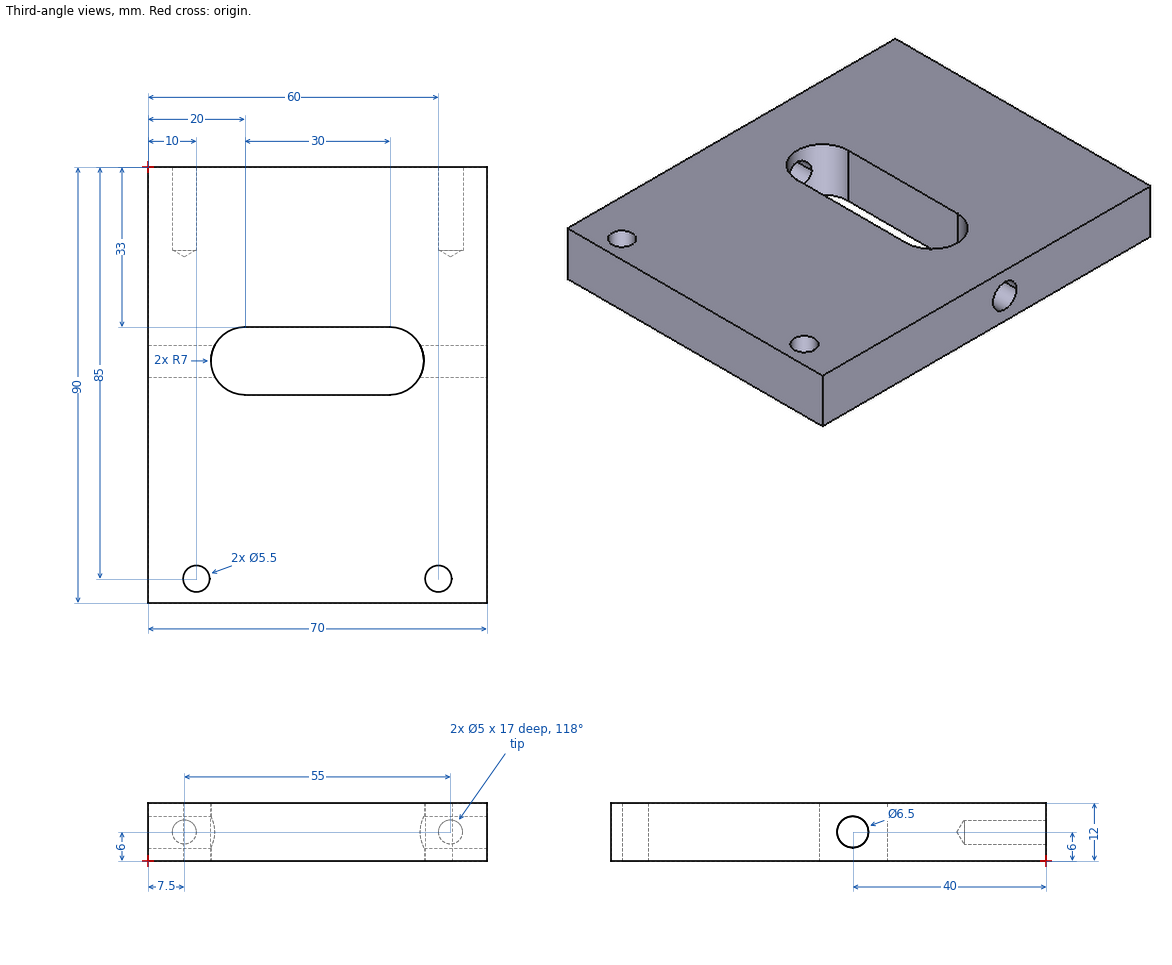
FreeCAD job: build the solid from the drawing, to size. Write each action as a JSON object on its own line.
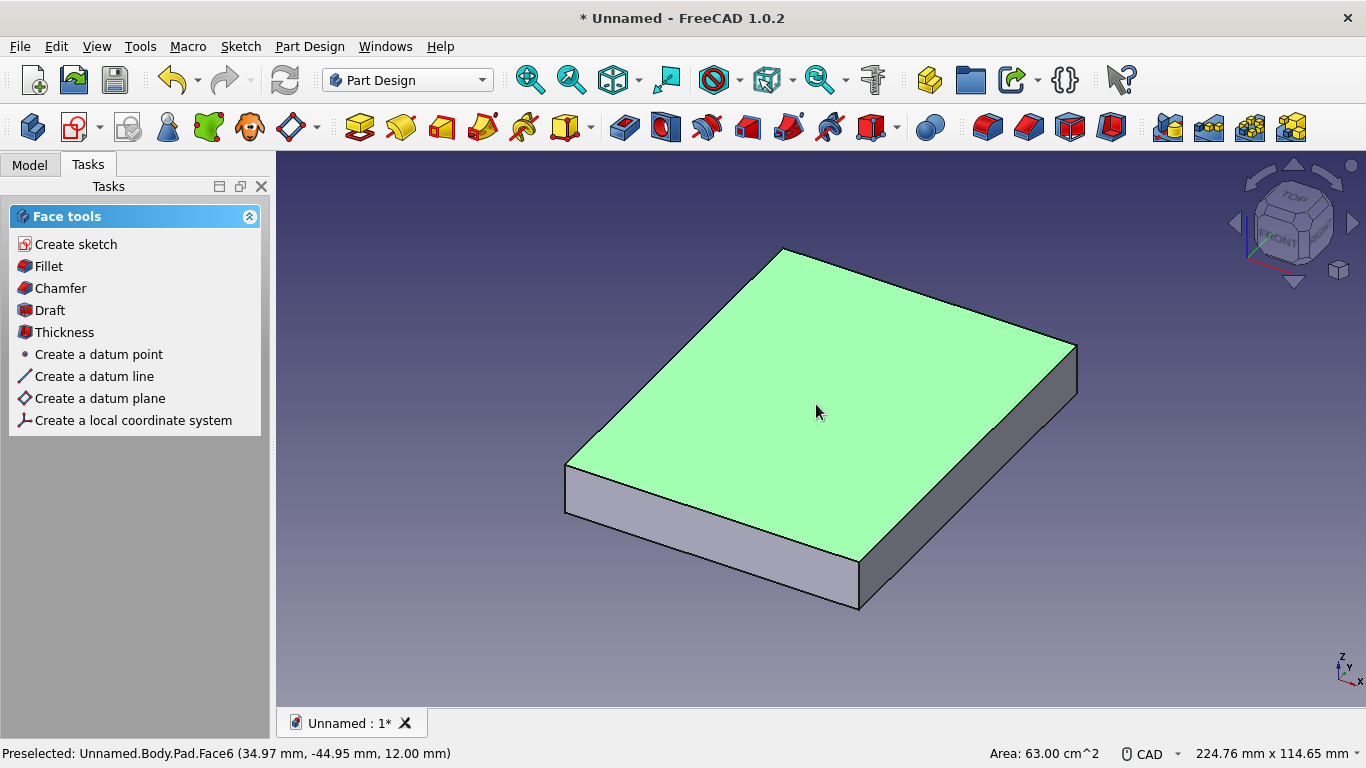
{"action": "left_click", "coordinate": [74, 128]}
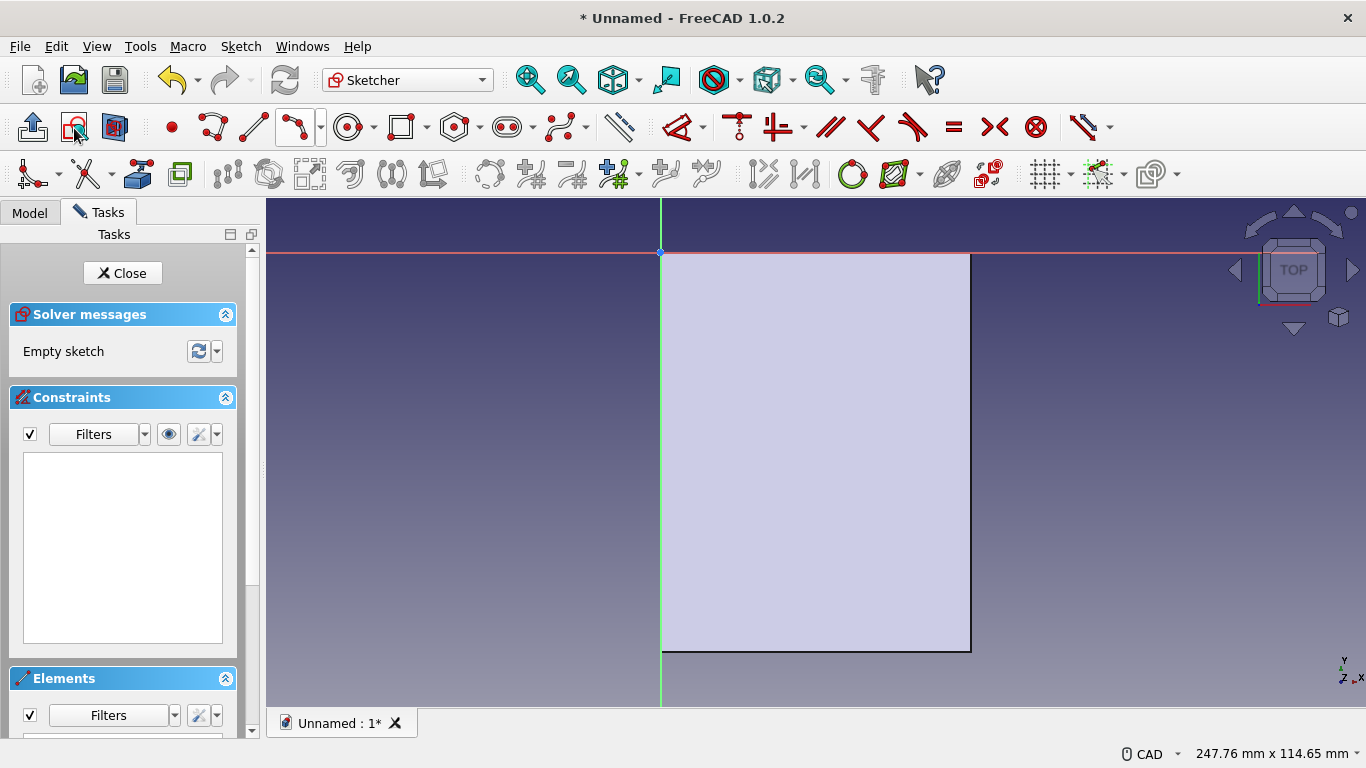
{"action": "scroll", "coordinate": [868, 226], "scroll_direction": "up", "scroll_amount": 2}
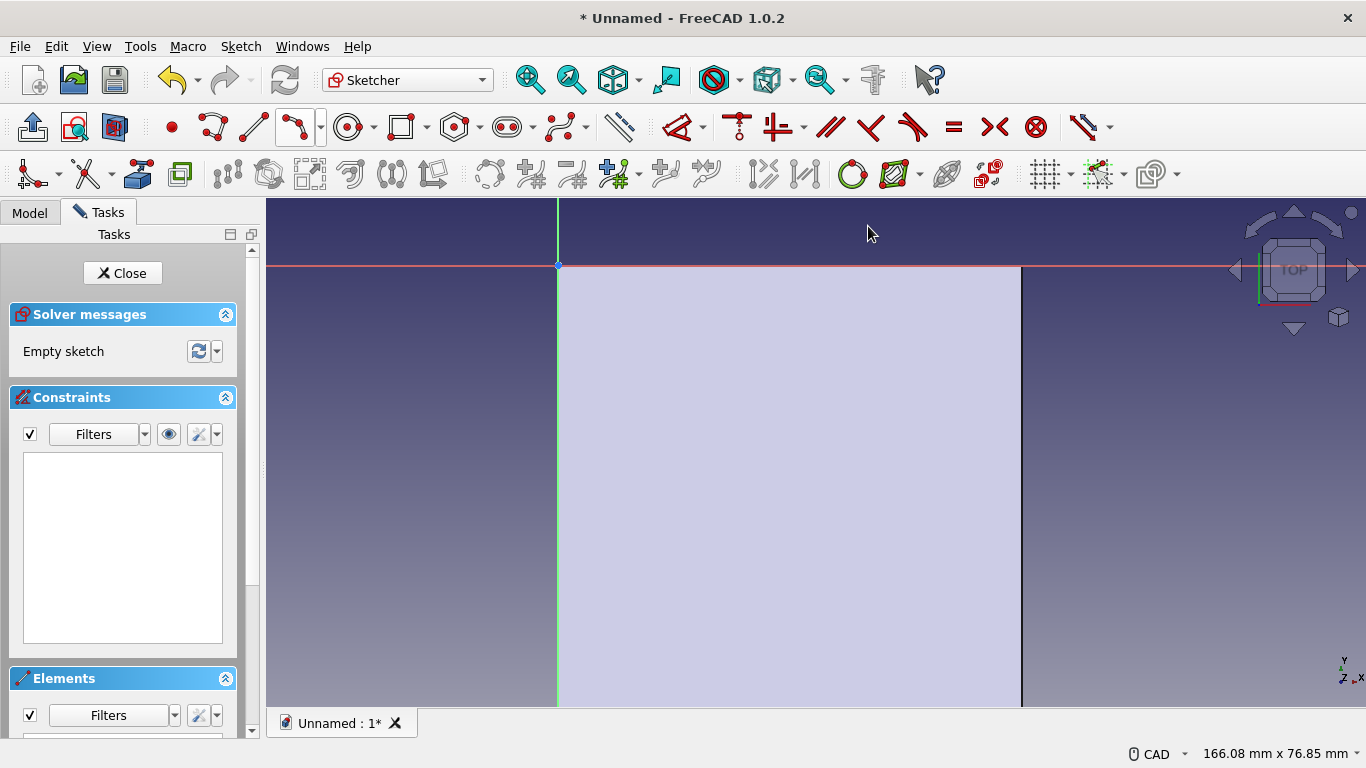
{"action": "left_click", "coordinate": [506, 128]}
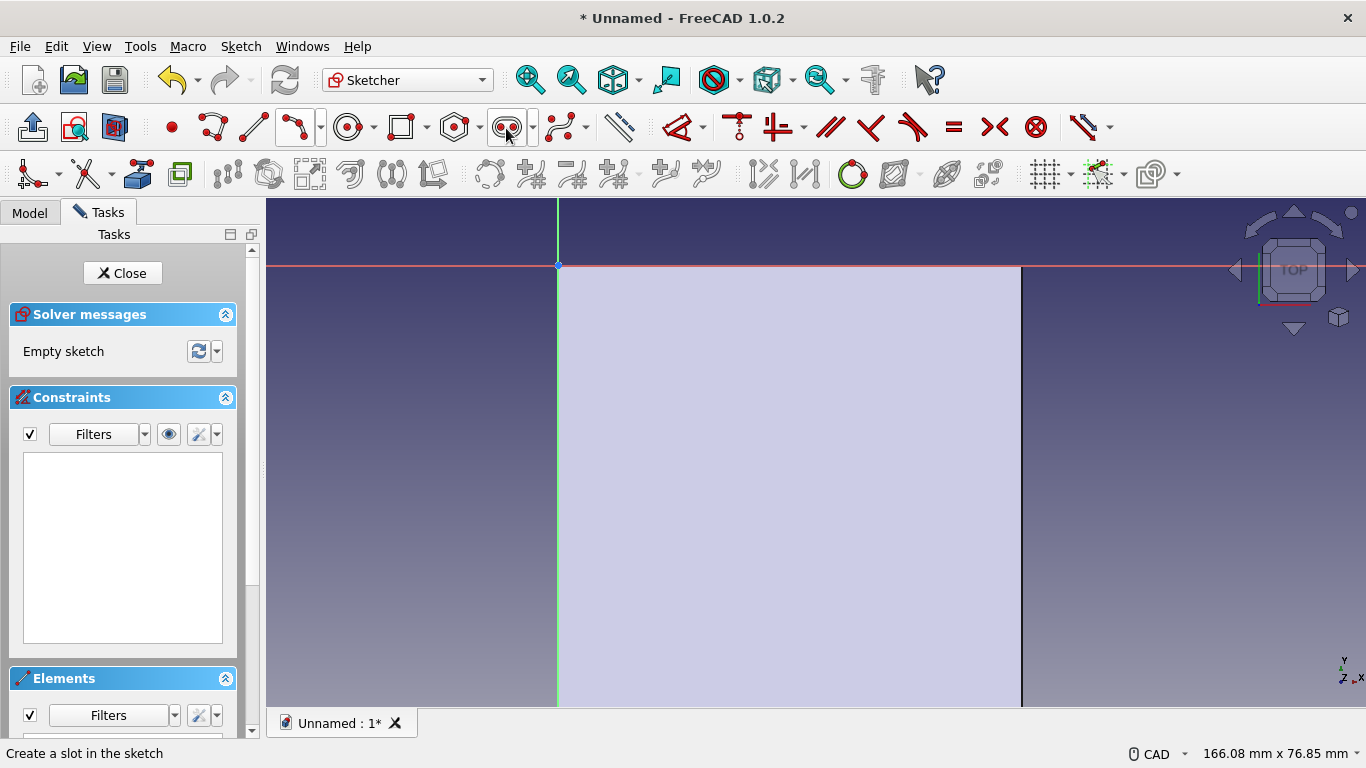
{"action": "left_click", "coordinate": [691, 531]}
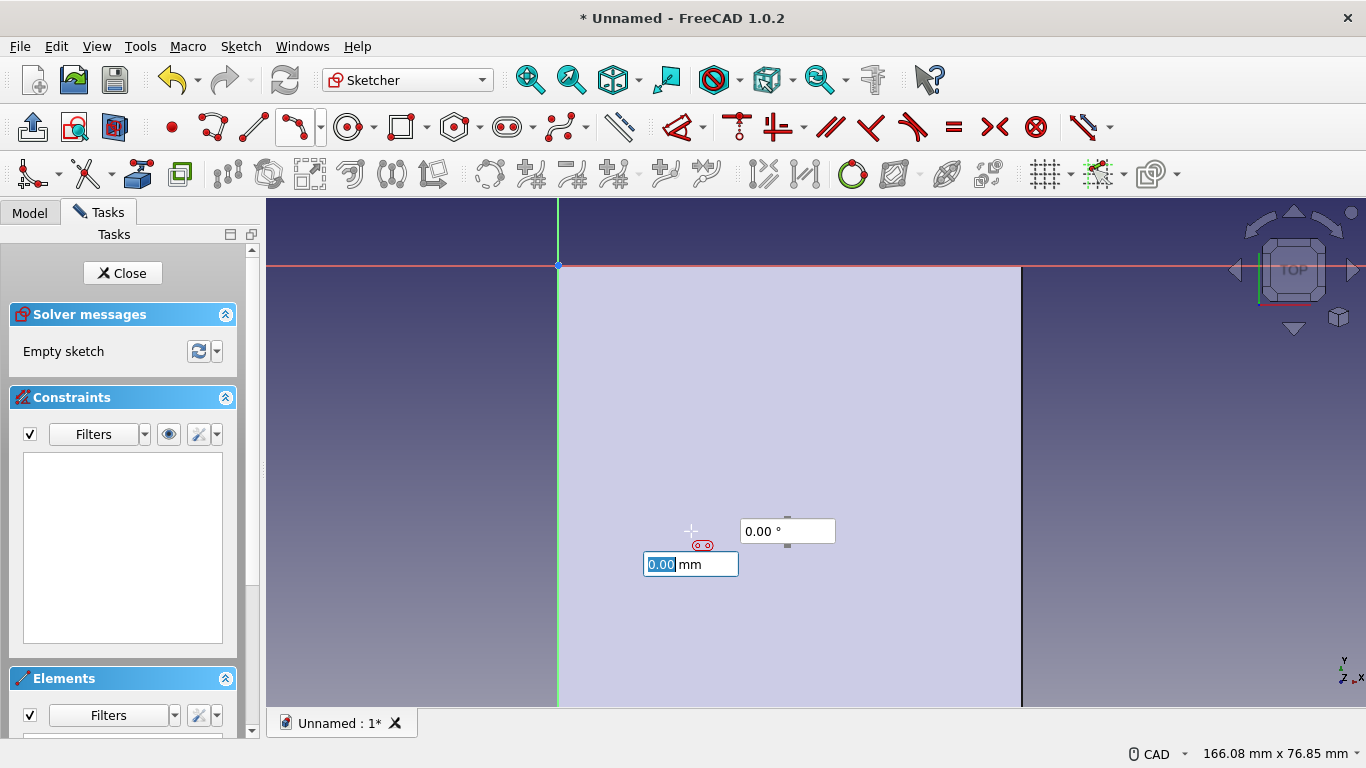
{"action": "left_click", "coordinate": [890, 531]}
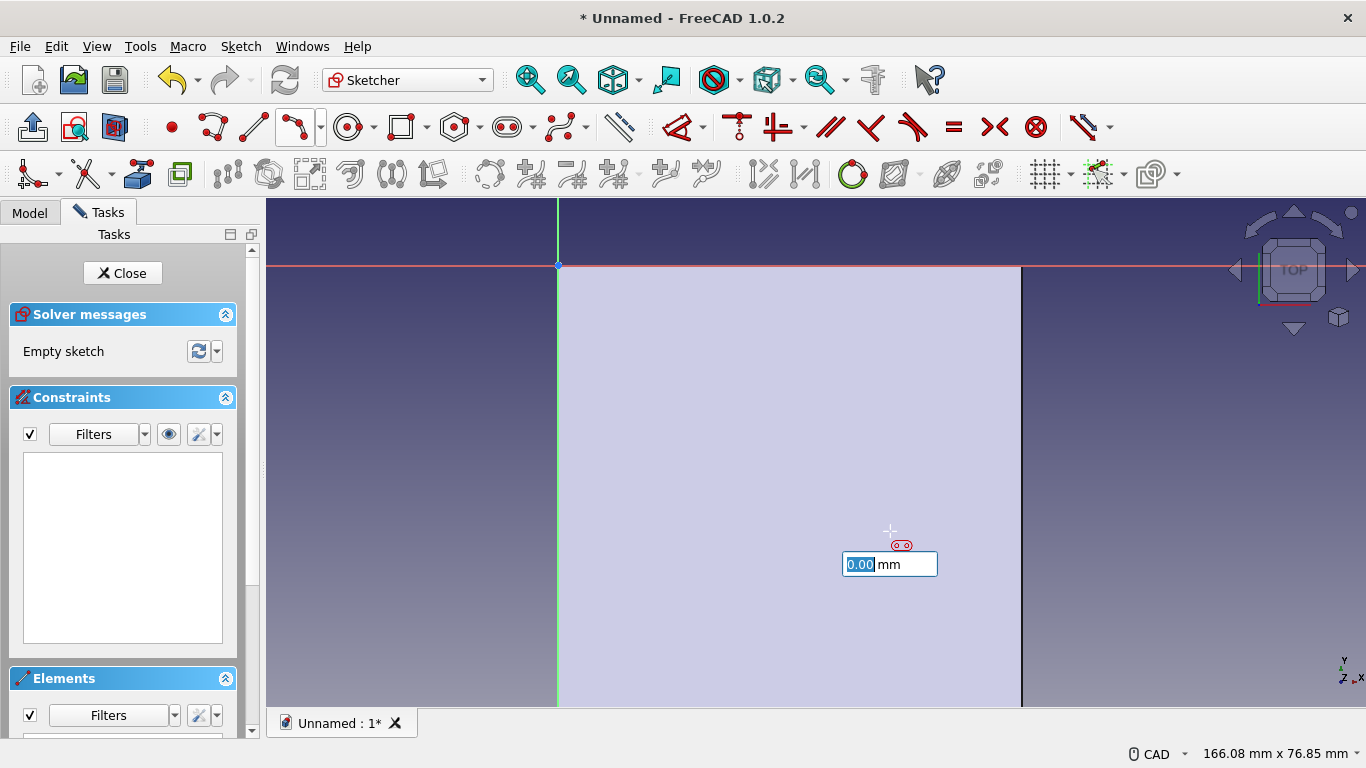
{"action": "left_click", "coordinate": [790, 484]}
{"action": "key", "text": "Escape"}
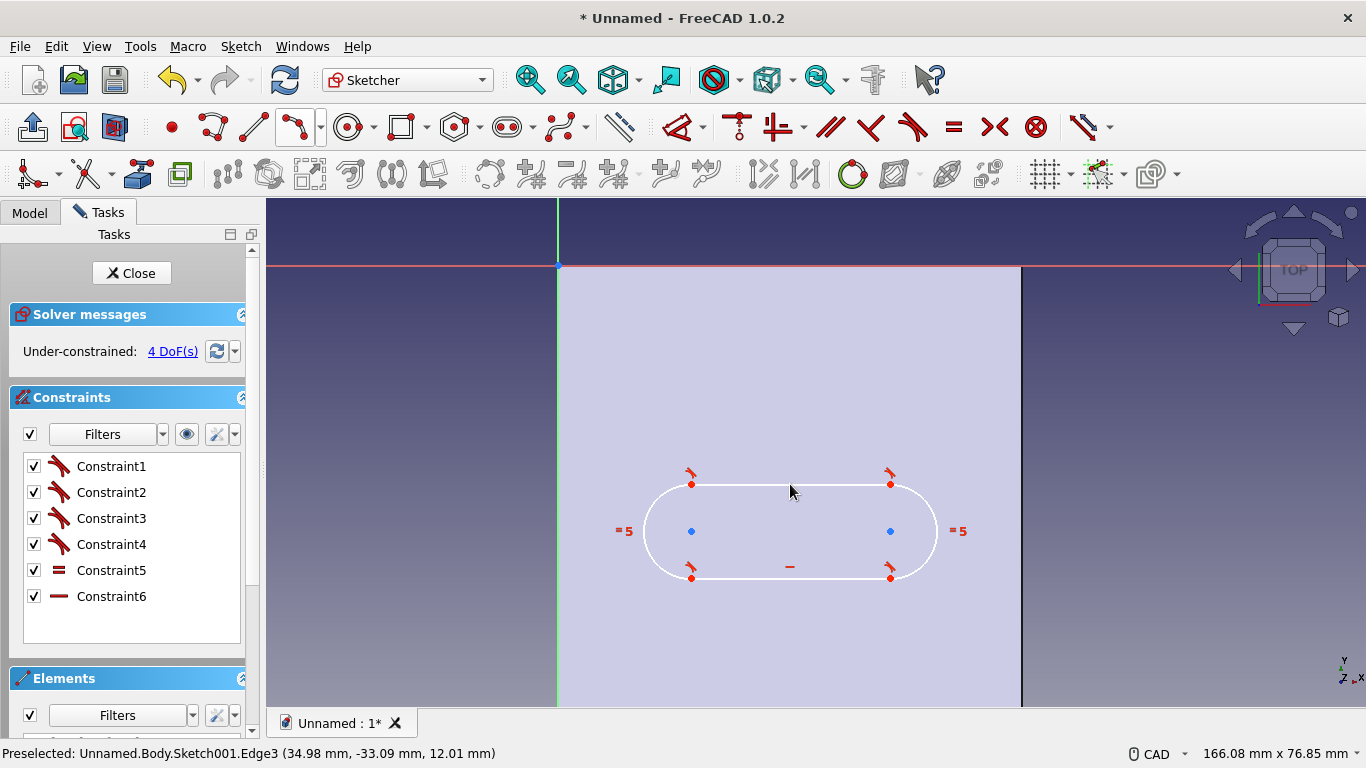
{"action": "left_click", "coordinate": [676, 128]}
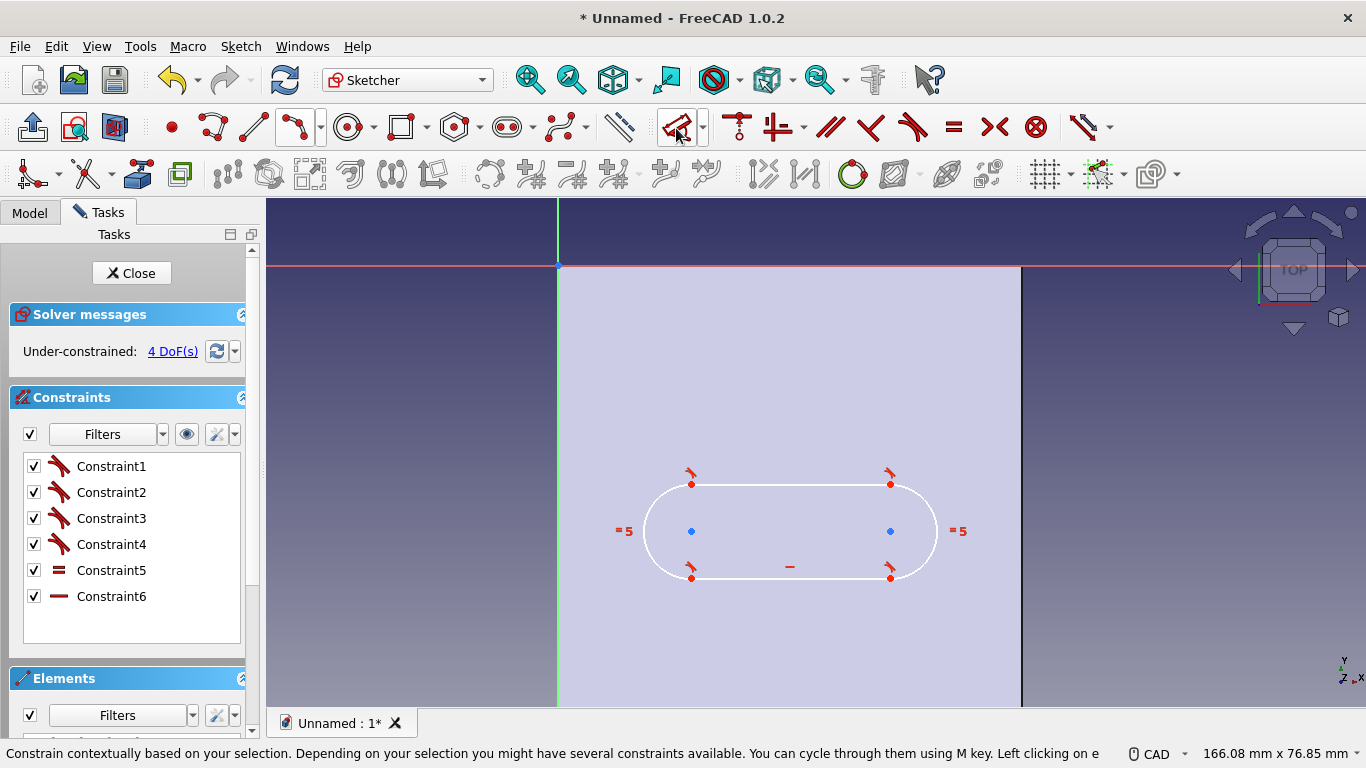
{"action": "left_click", "coordinate": [653, 504]}
{"action": "left_click", "coordinate": [627, 485]}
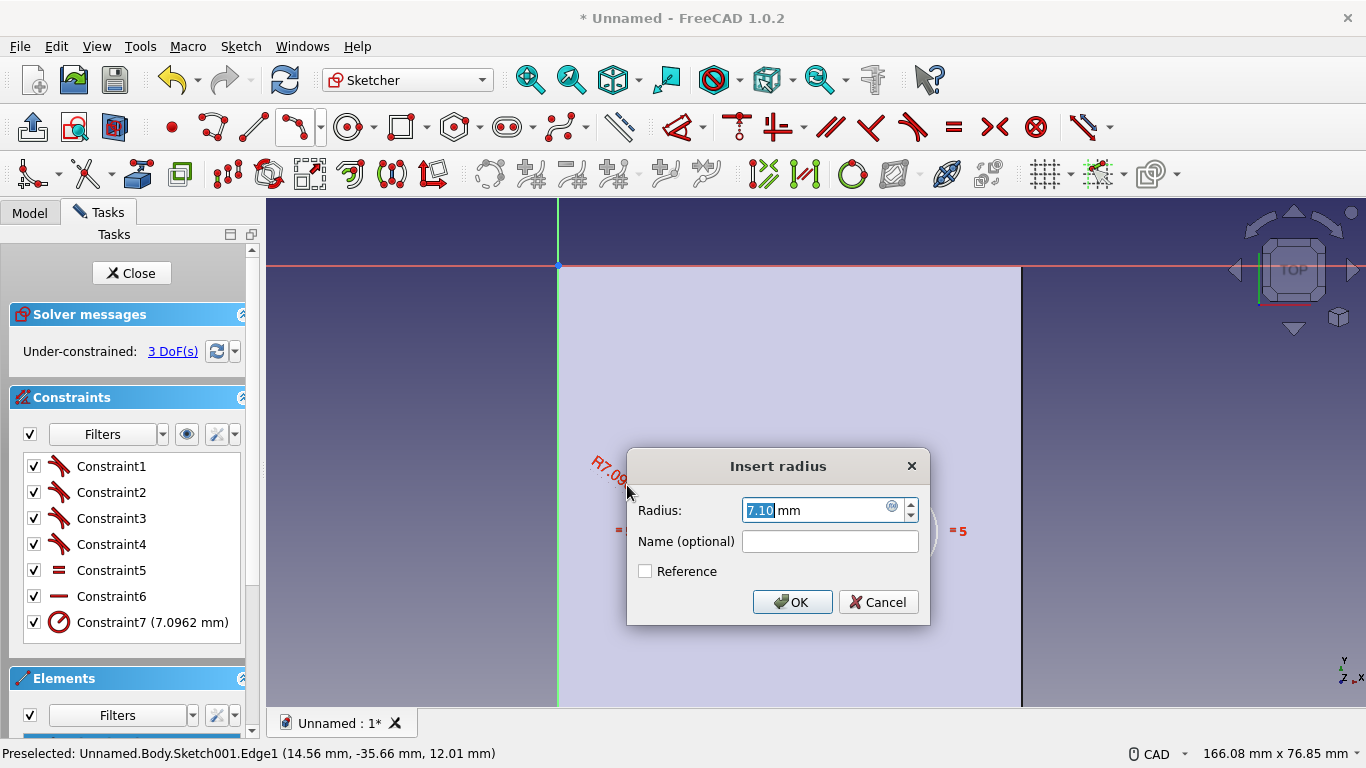
{"action": "type", "text": "7"}
{"action": "key", "text": "Return"}